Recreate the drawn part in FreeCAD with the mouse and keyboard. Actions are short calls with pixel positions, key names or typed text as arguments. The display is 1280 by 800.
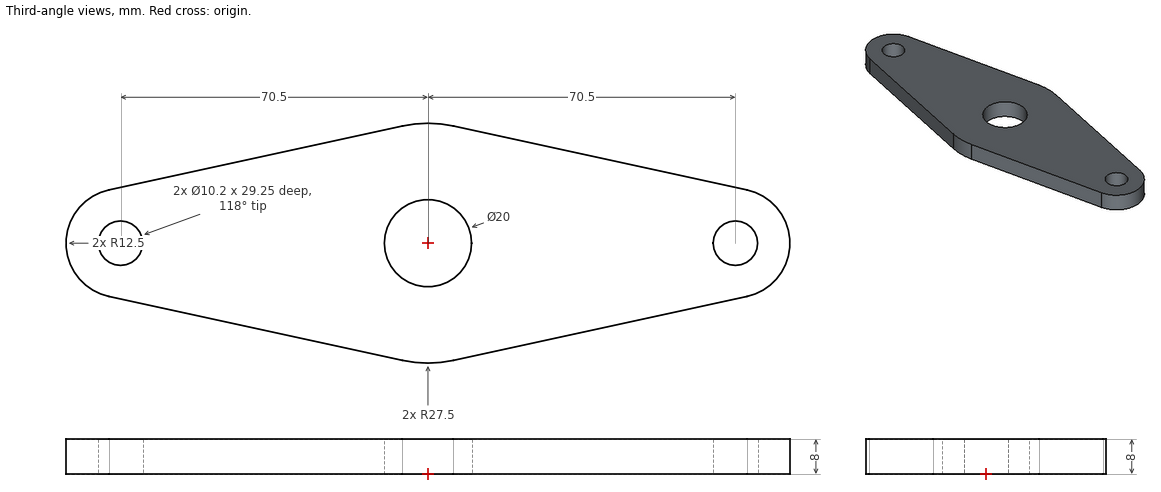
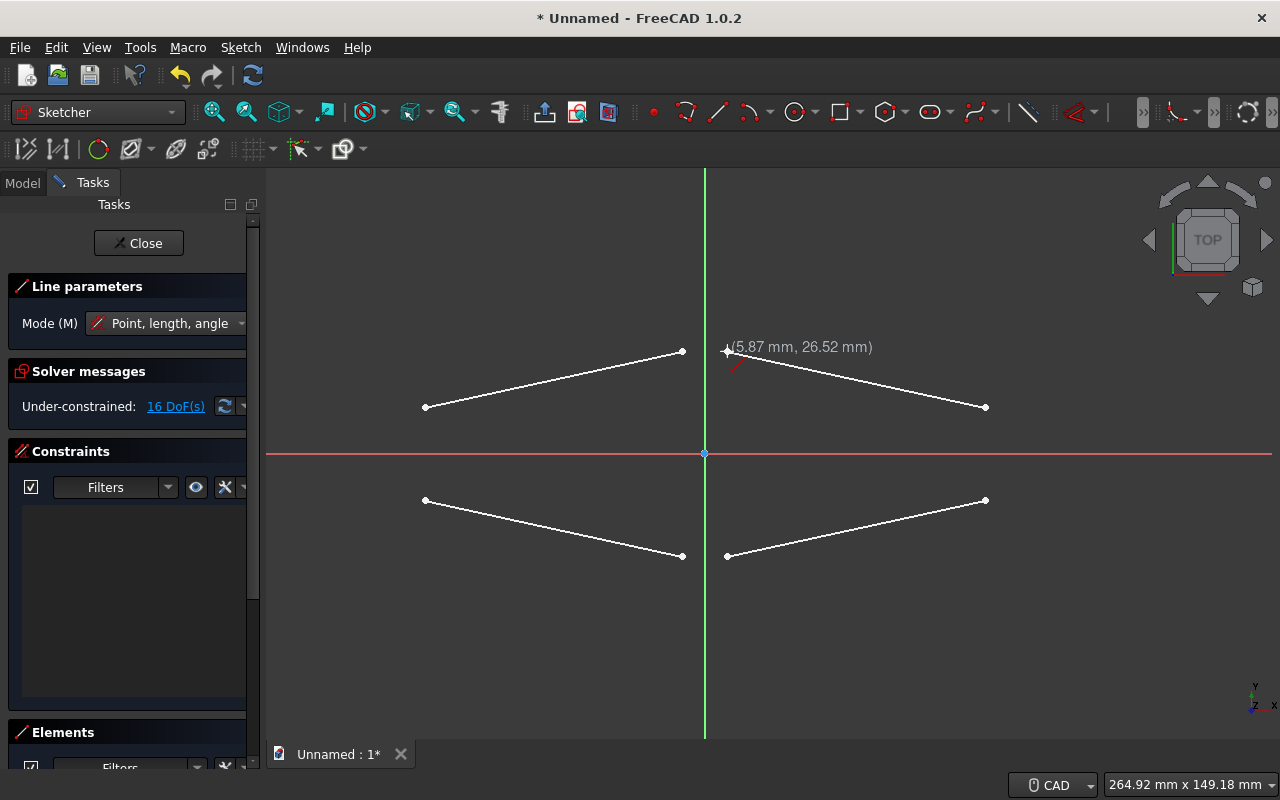
key(g)
key(3)
key(a)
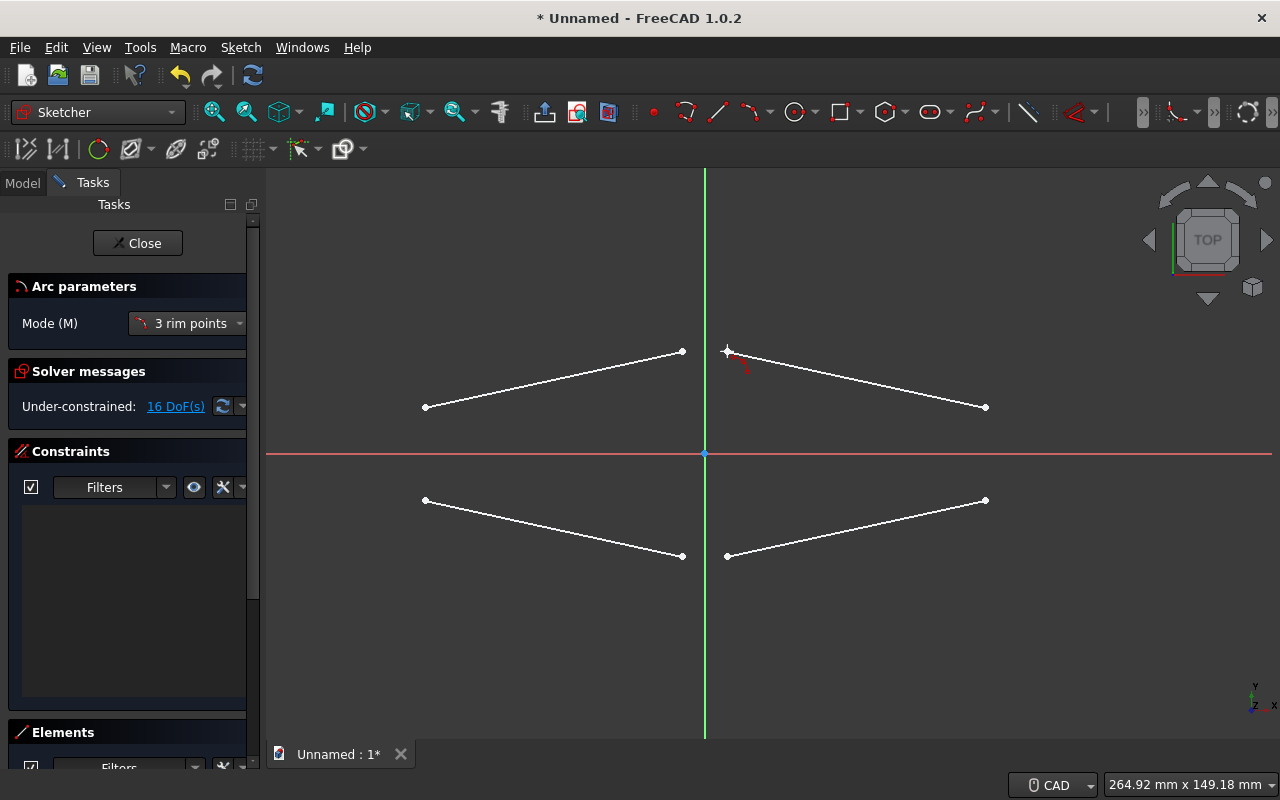
click(425, 408)
click(425, 501)
click(394, 429)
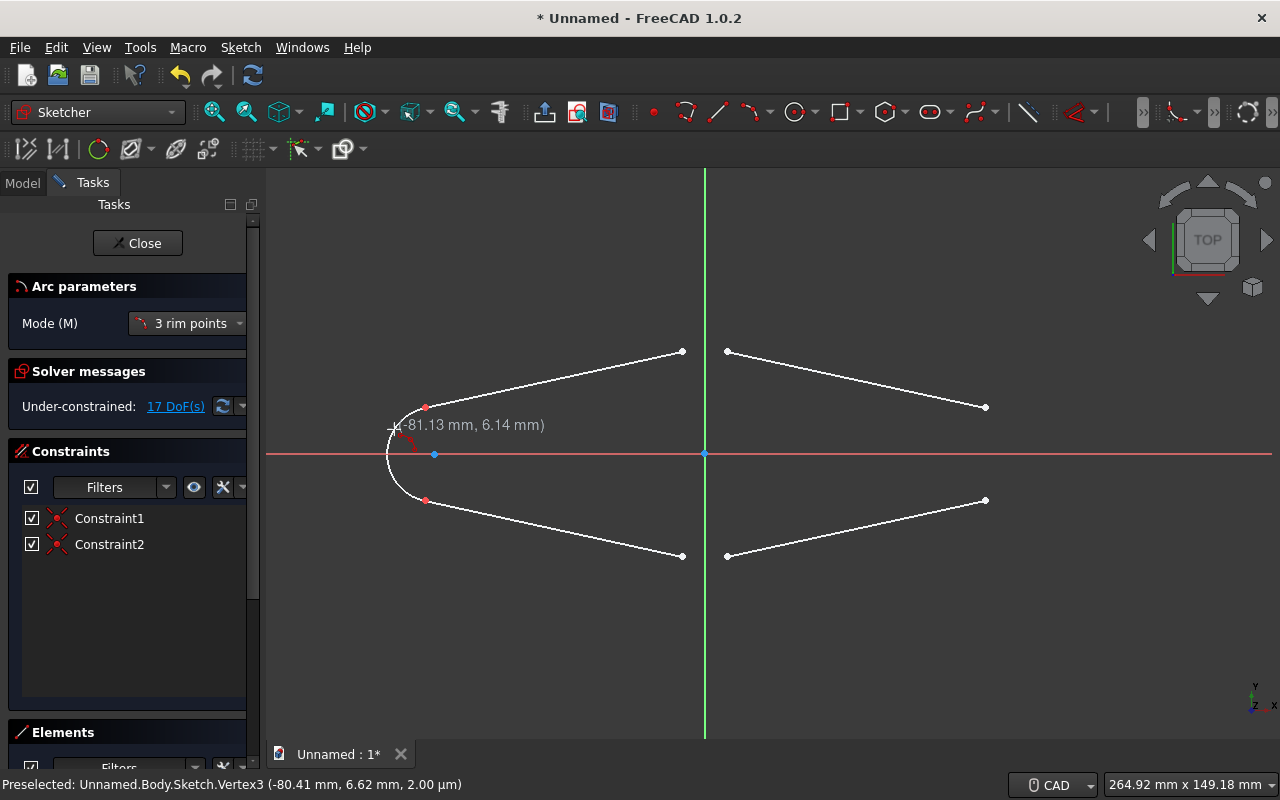
click(682, 557)
click(727, 557)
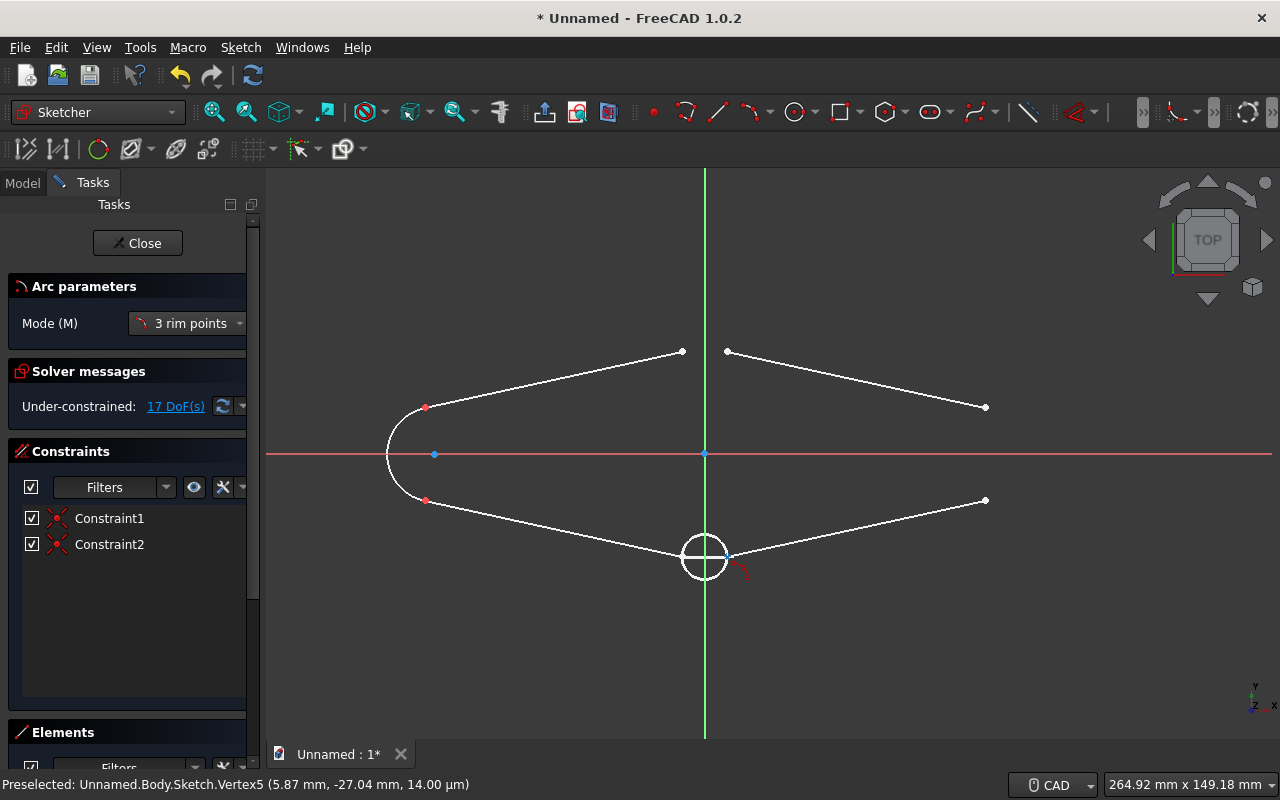
scroll(700, 559, up, 10)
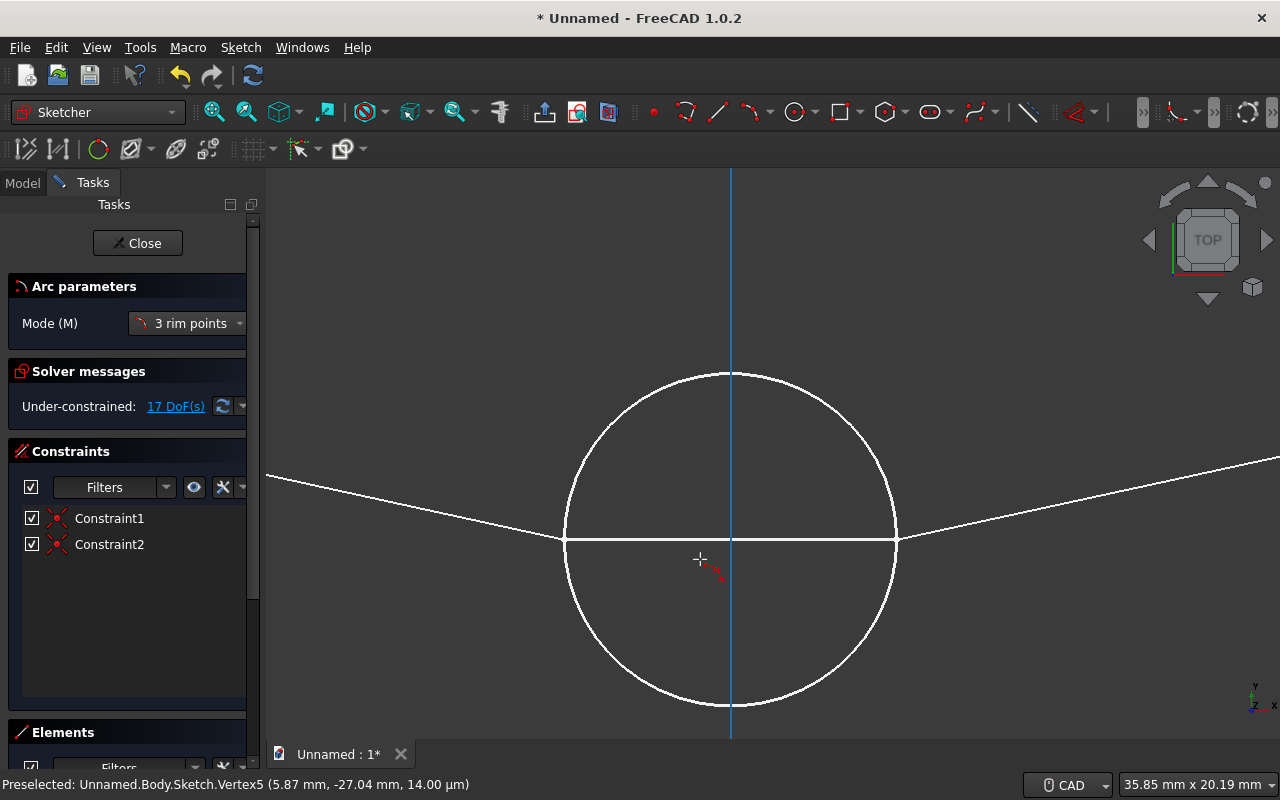
click(697, 552)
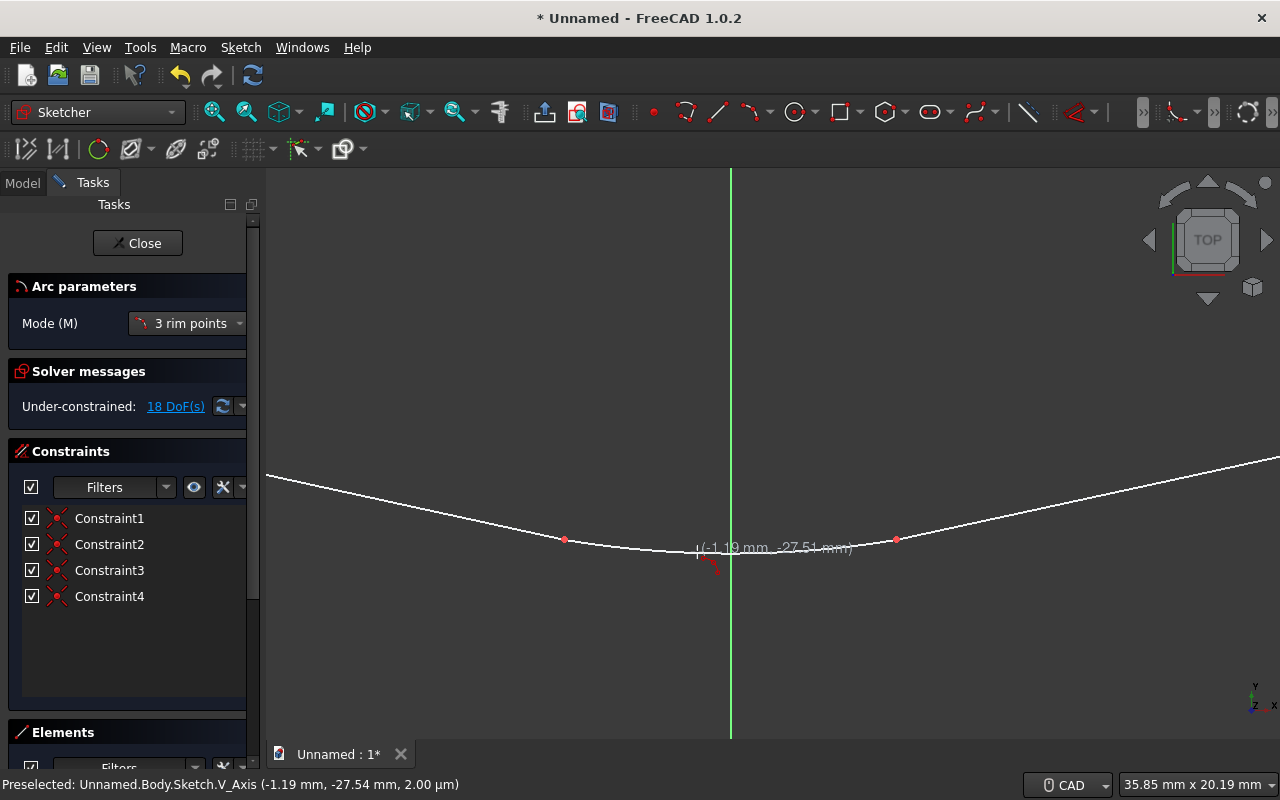
scroll(700, 560, down, 10)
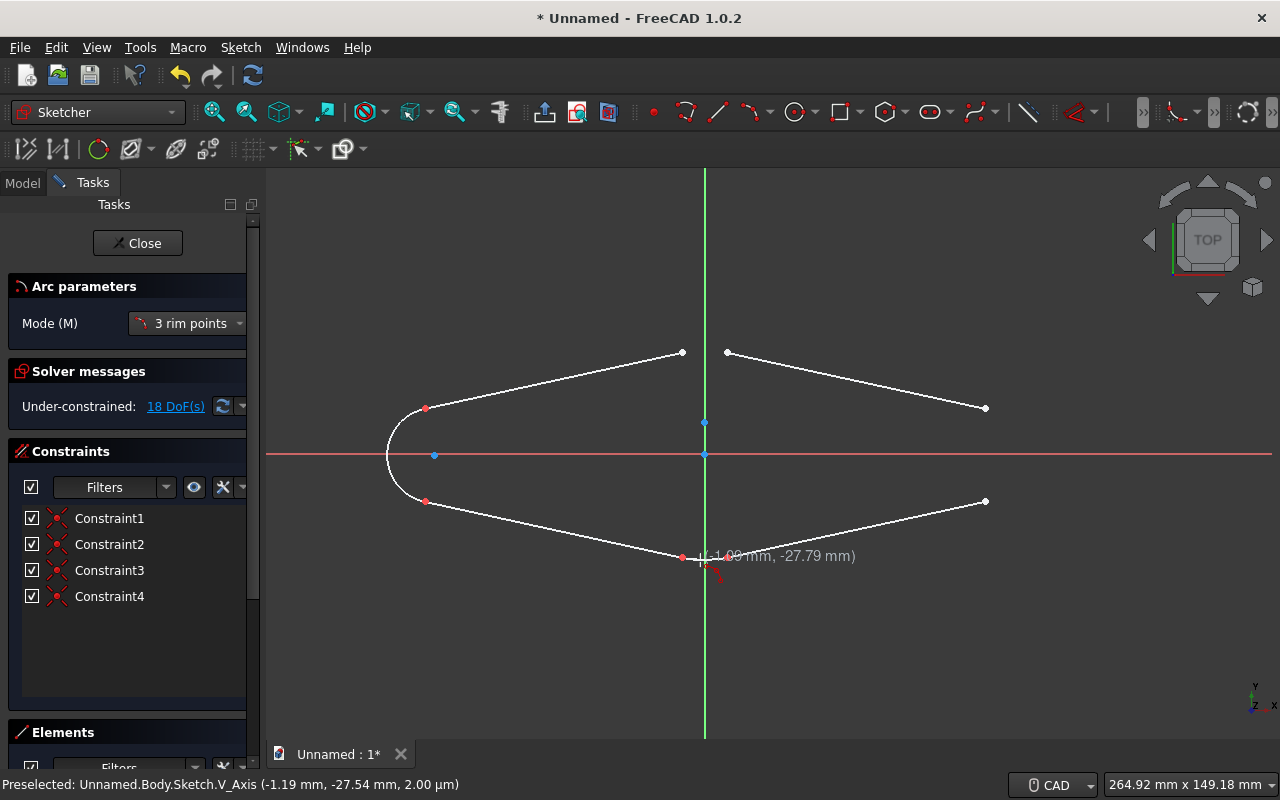
click(985, 502)
click(985, 409)
click(1015, 479)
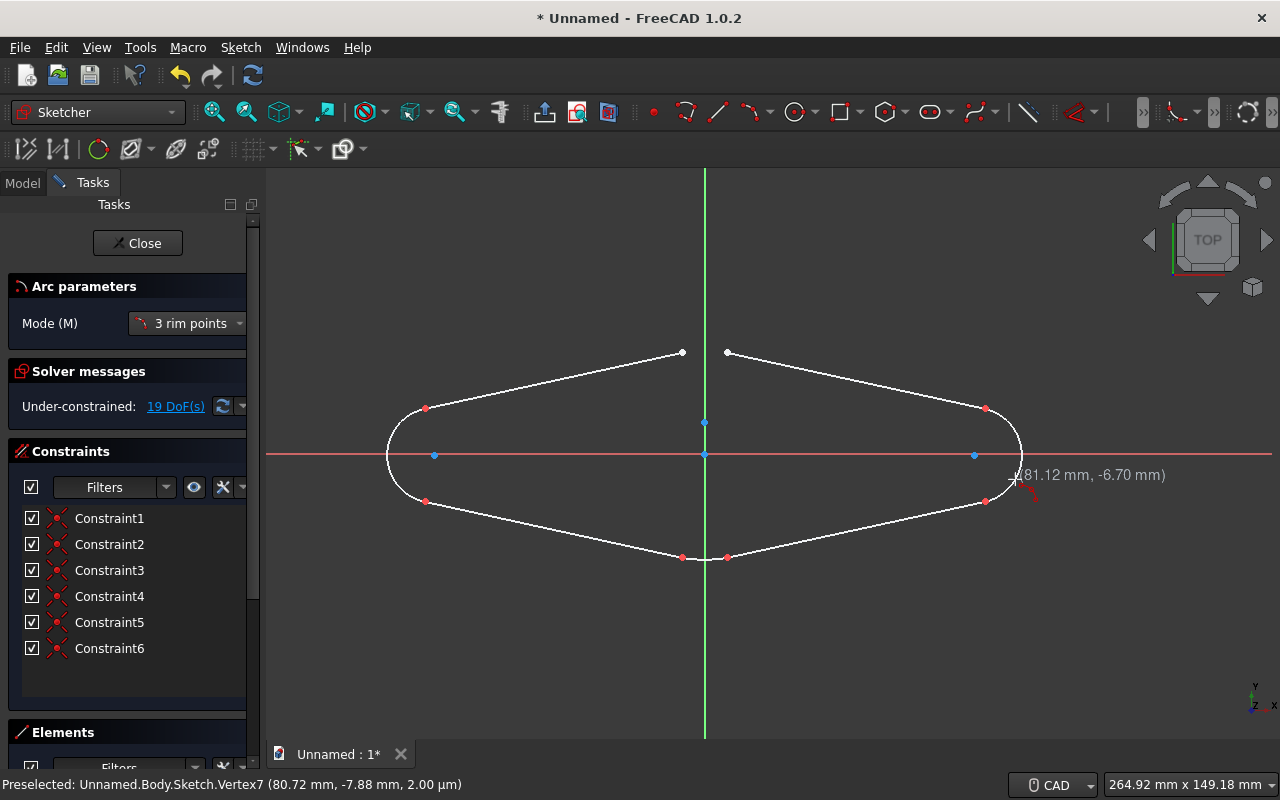
click(727, 353)
click(682, 353)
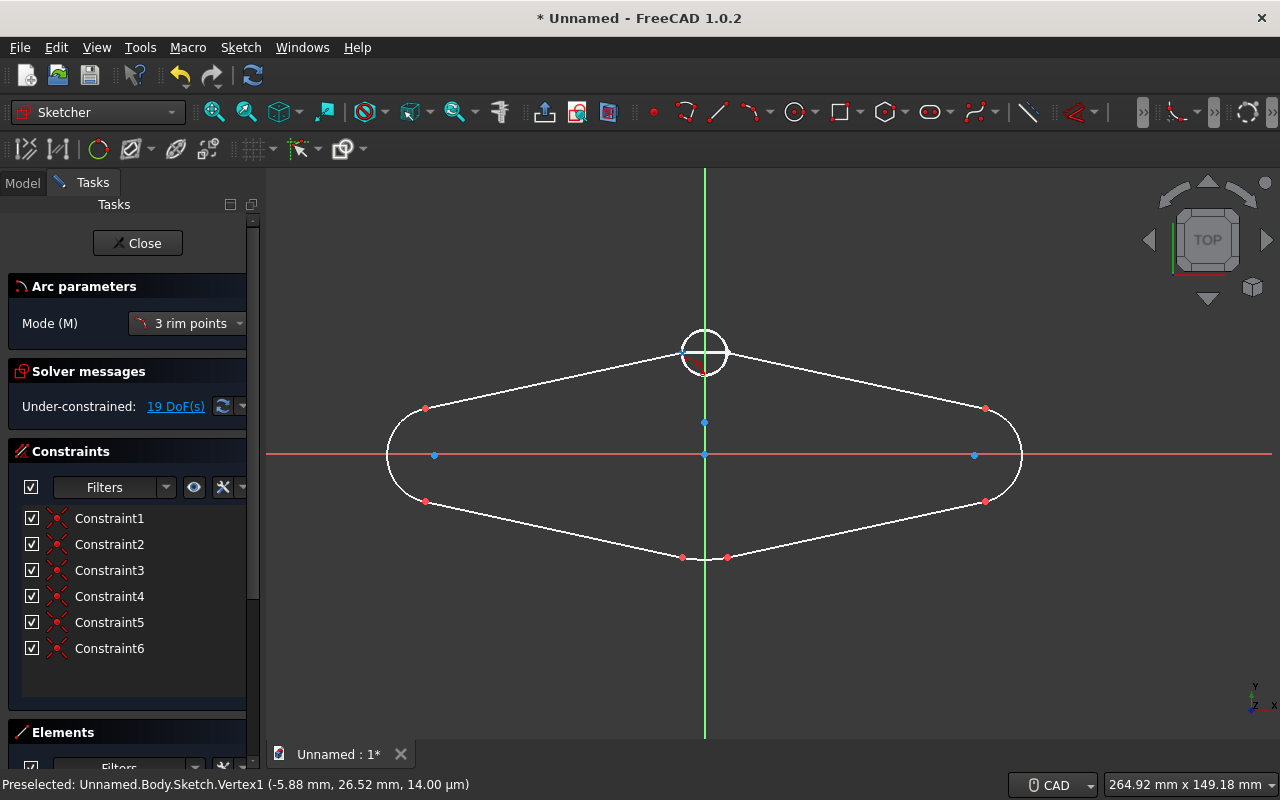
scroll(709, 349, up, 10)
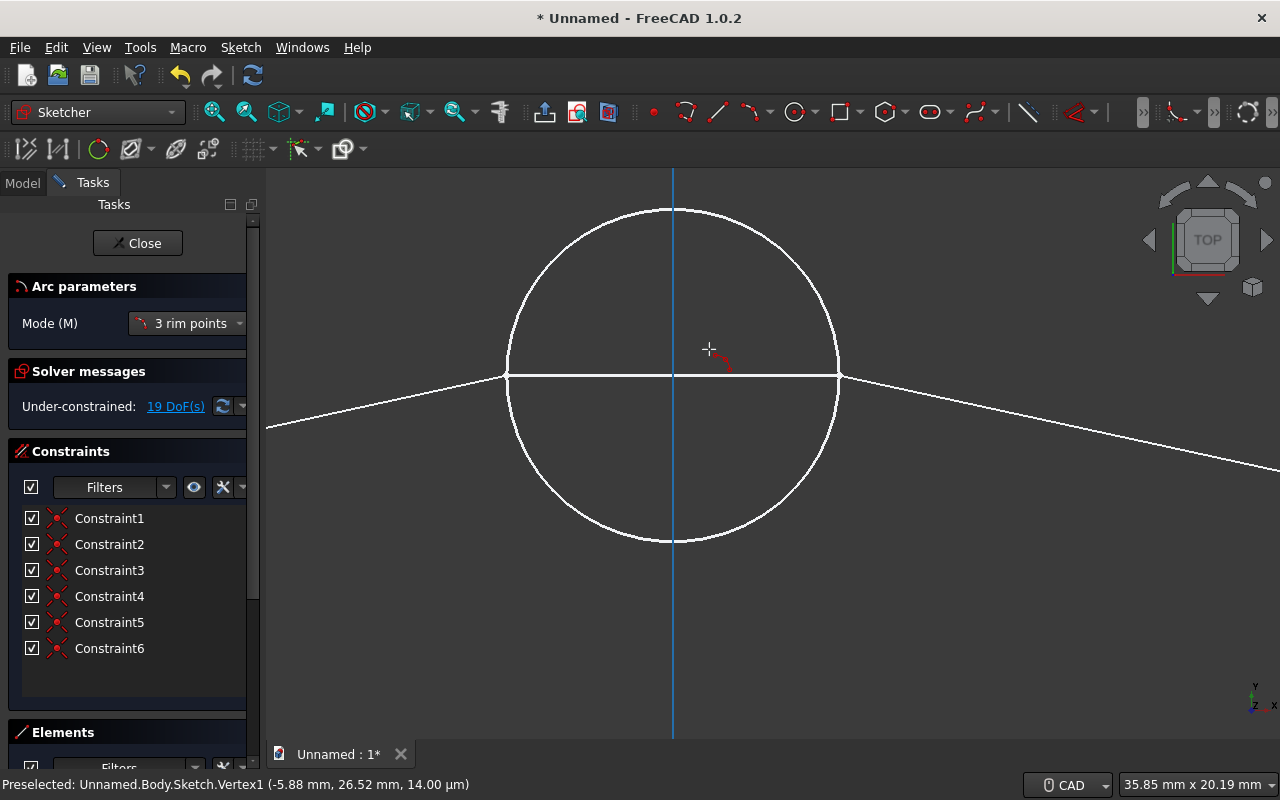
click(706, 348)
key(Escape)